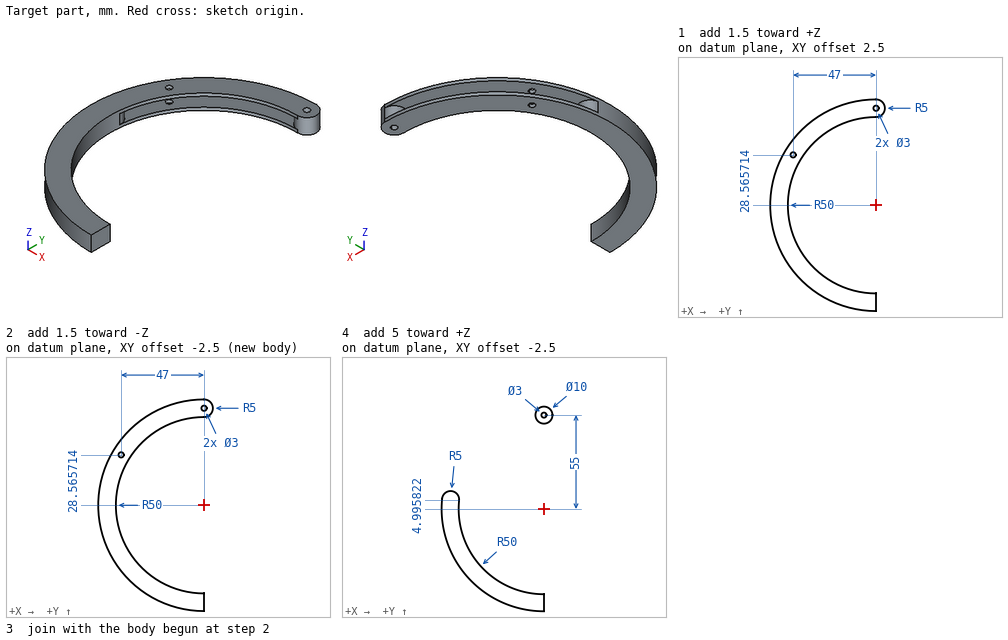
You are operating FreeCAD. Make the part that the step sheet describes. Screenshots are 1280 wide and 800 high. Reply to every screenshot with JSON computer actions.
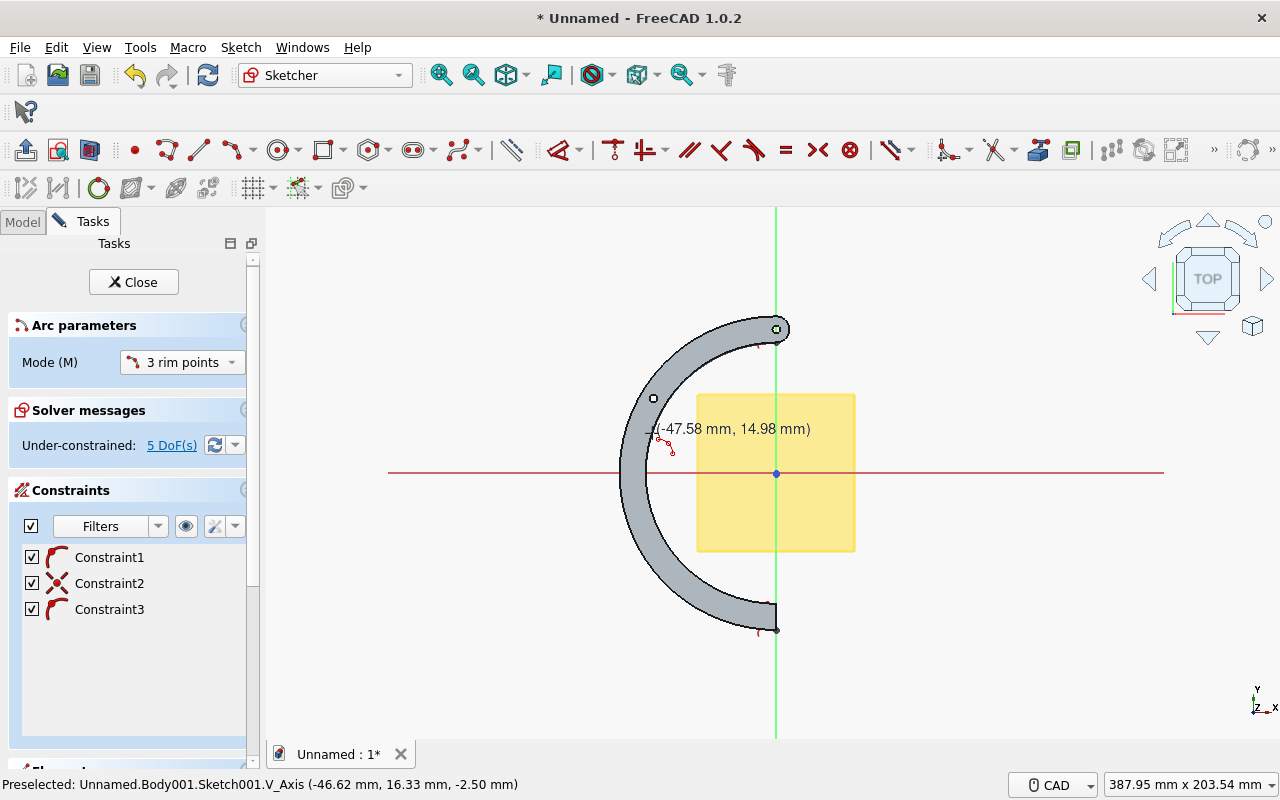
{"action": "left_click", "coordinate": [776, 343]}
{"action": "left_click", "coordinate": [776, 316]}
{"action": "left_click", "coordinate": [789, 329]}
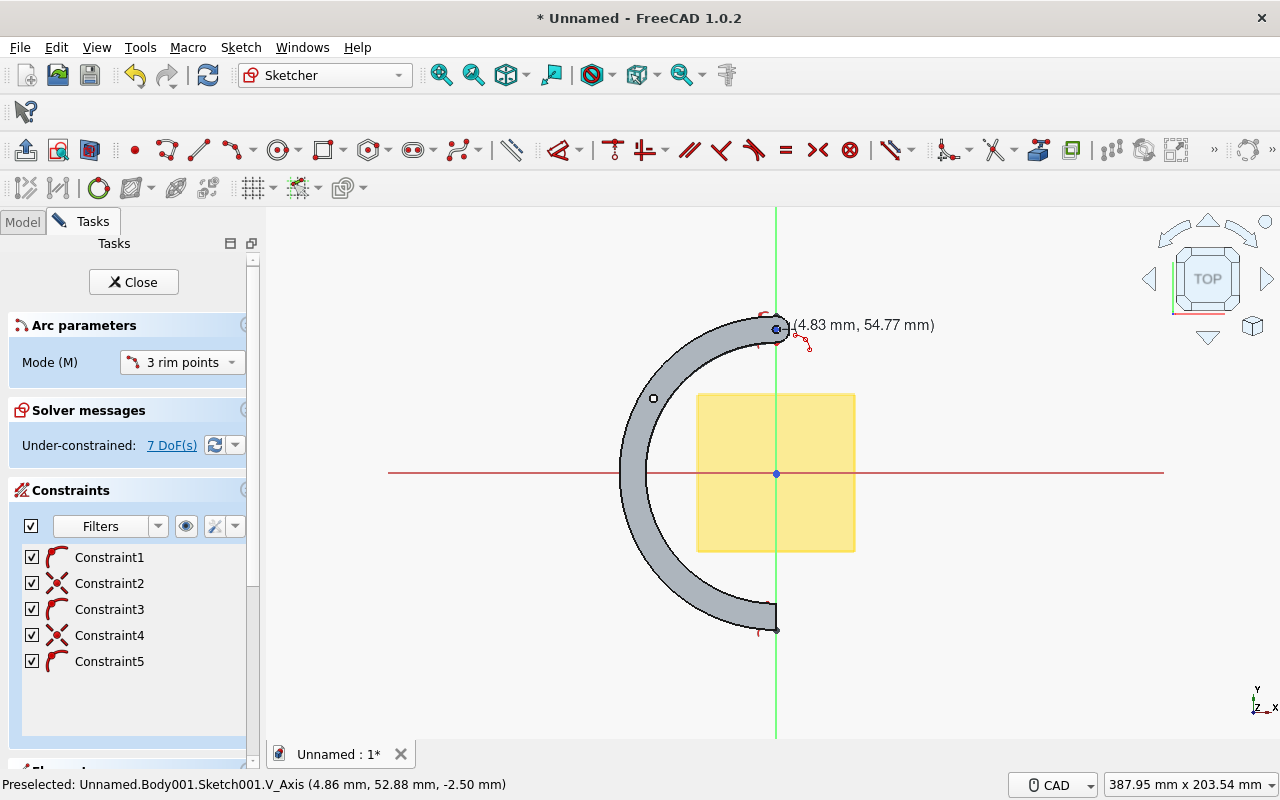
{"action": "left_click", "coordinate": [776, 317]}
{"action": "left_click", "coordinate": [776, 631]}
{"action": "left_click", "coordinate": [627, 425]}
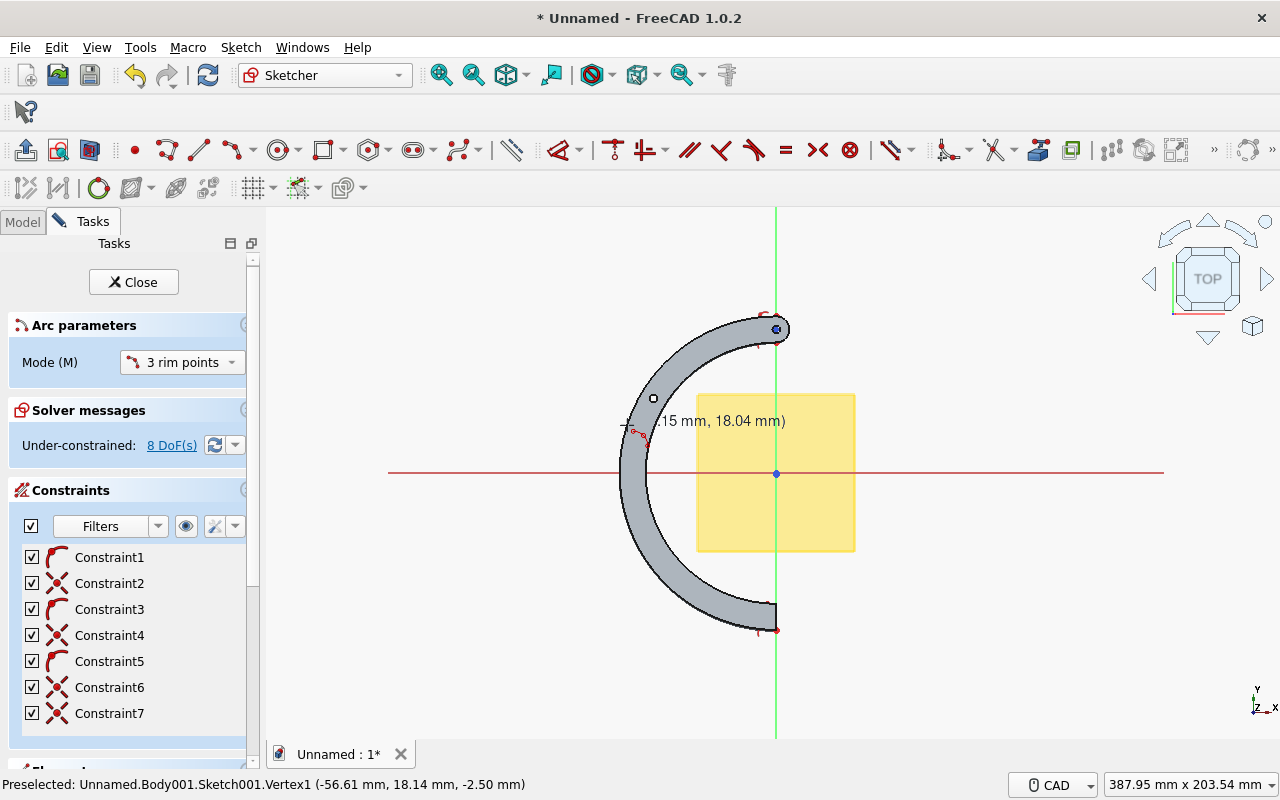
{"action": "left_click", "coordinate": [278, 150]}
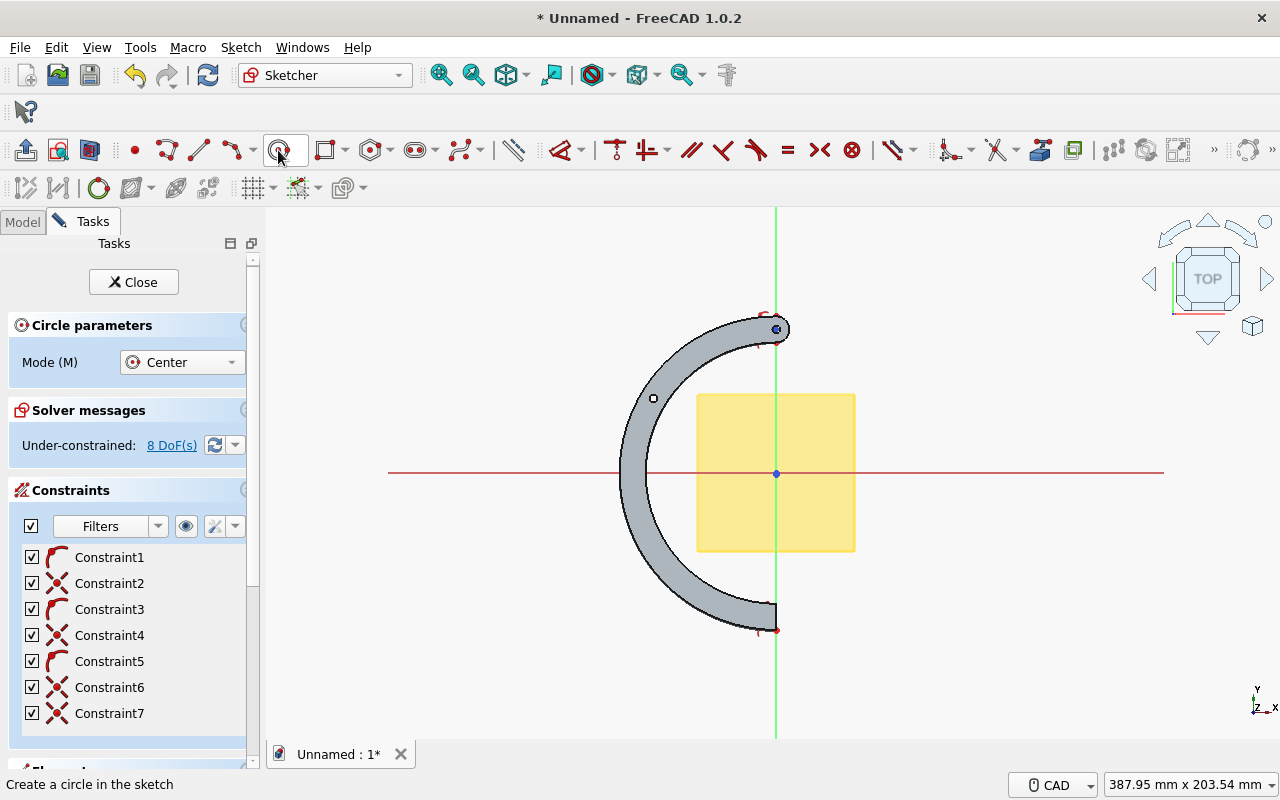
{"action": "scroll", "coordinate": [654, 399], "scroll_direction": "up", "scroll_amount": 9}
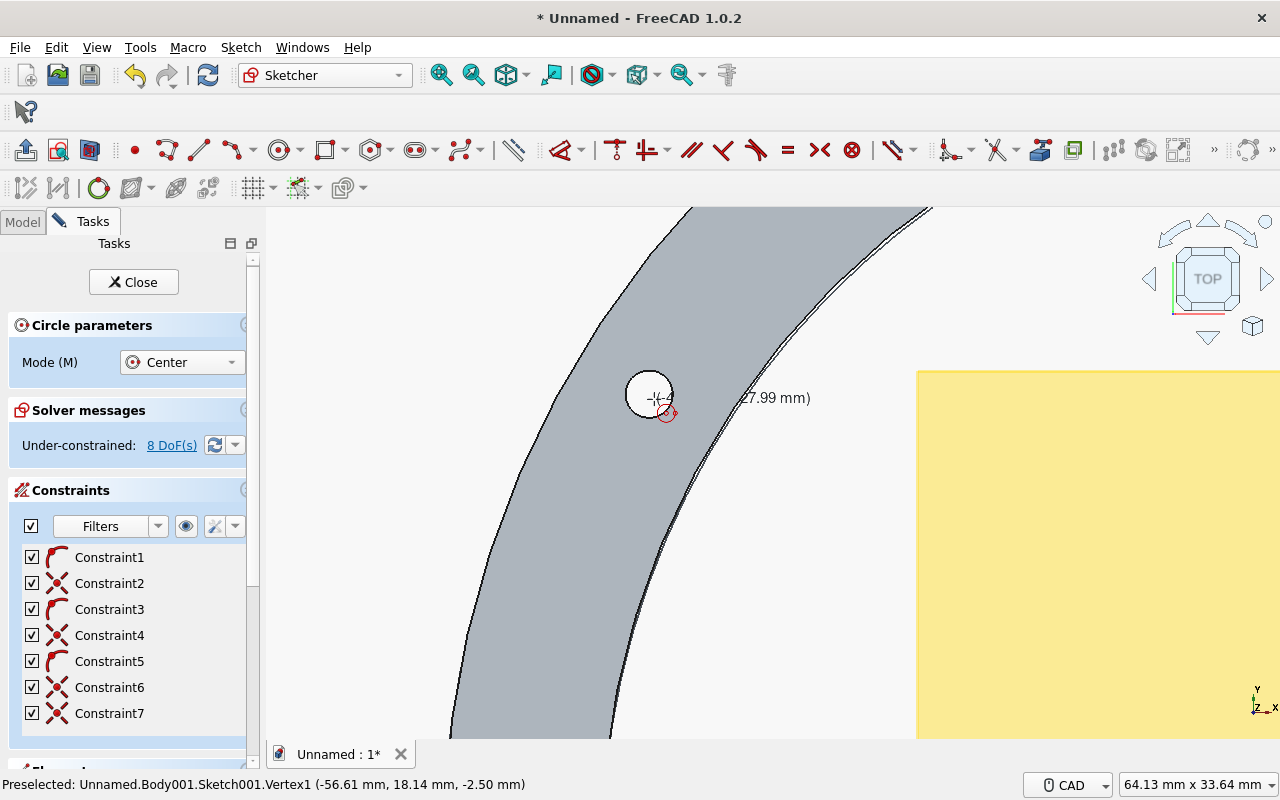
{"action": "scroll", "coordinate": [654, 399], "scroll_direction": "down", "scroll_amount": 9}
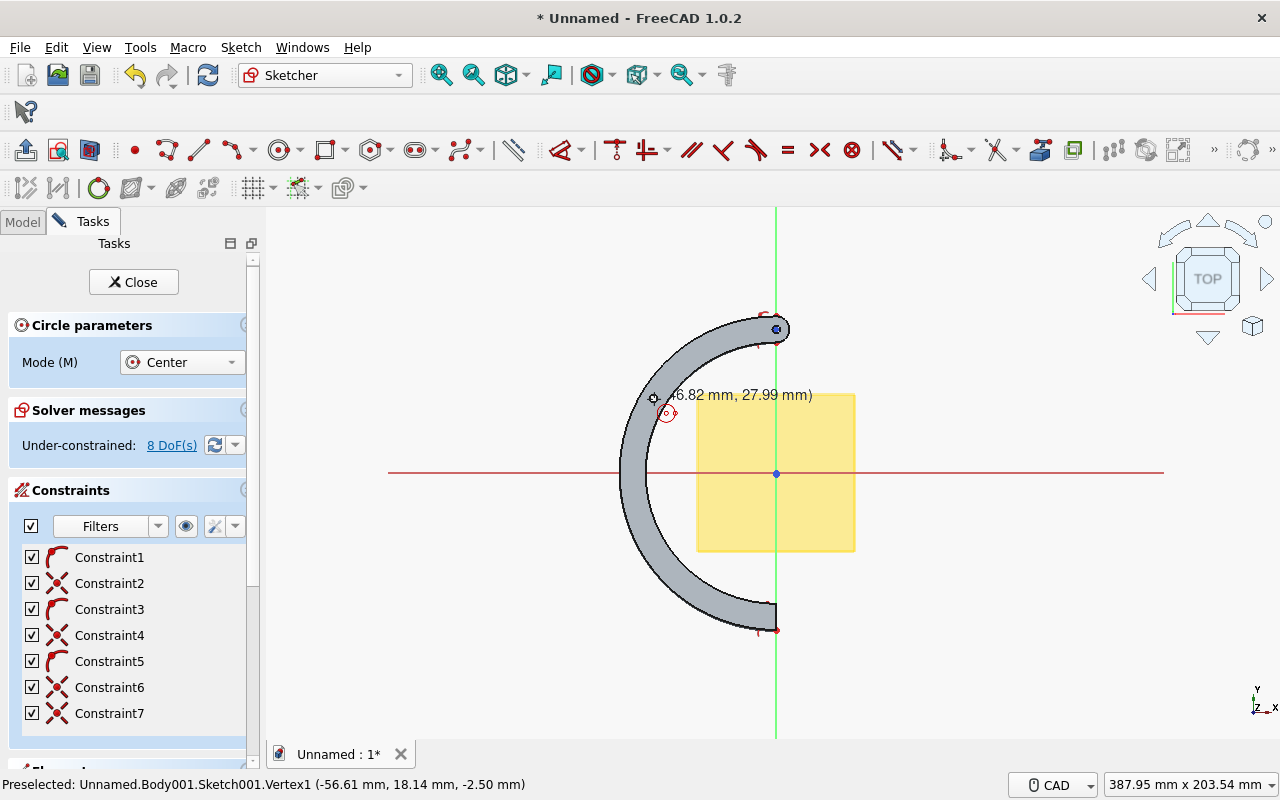
{"action": "left_click", "coordinate": [654, 399]}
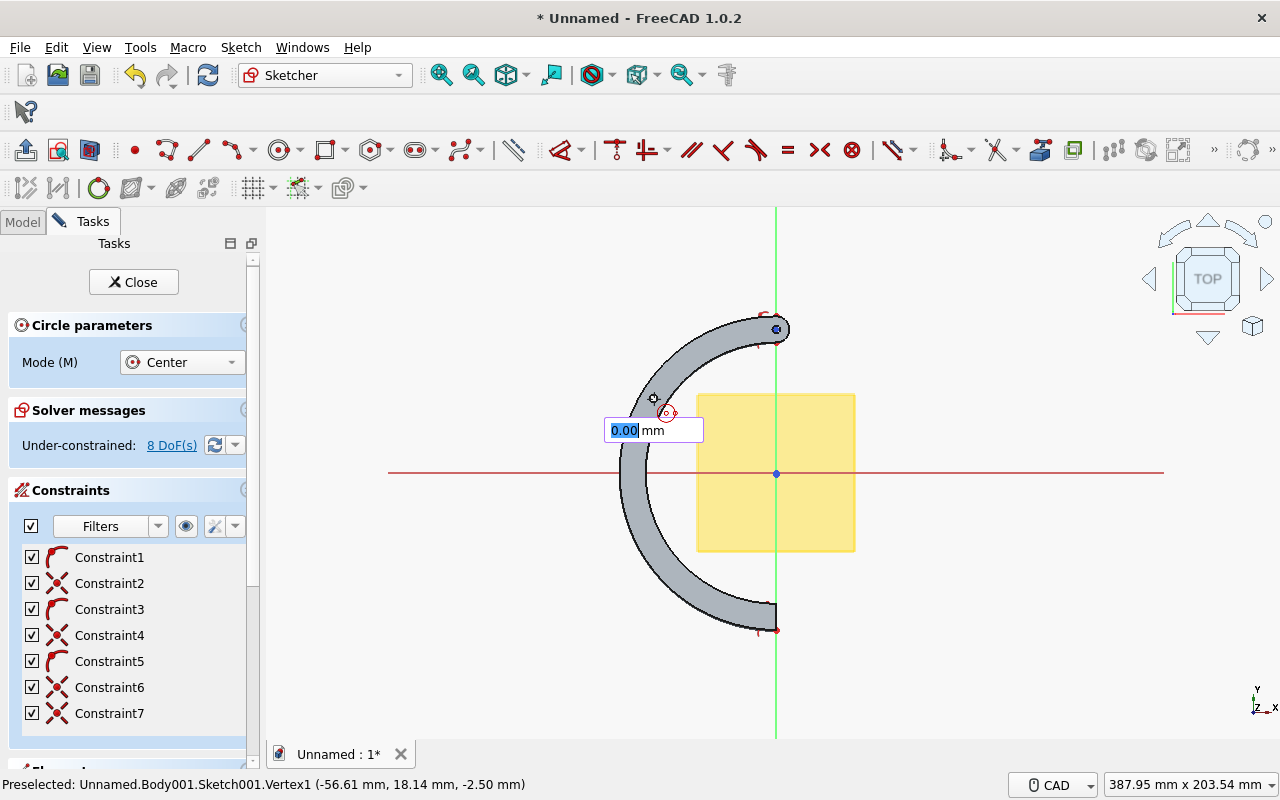
{"action": "scroll", "coordinate": [652, 402], "scroll_direction": "up", "scroll_amount": 7}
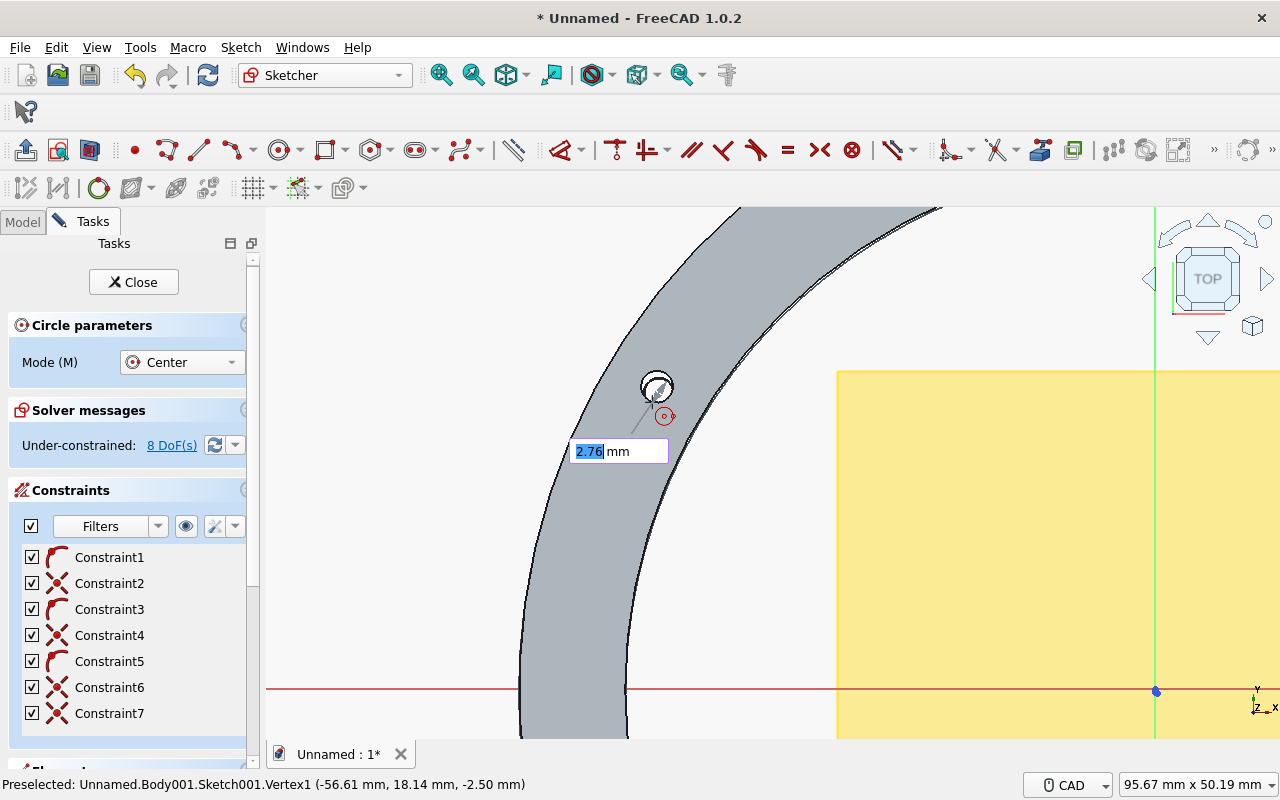
{"action": "left_click", "coordinate": [652, 402]}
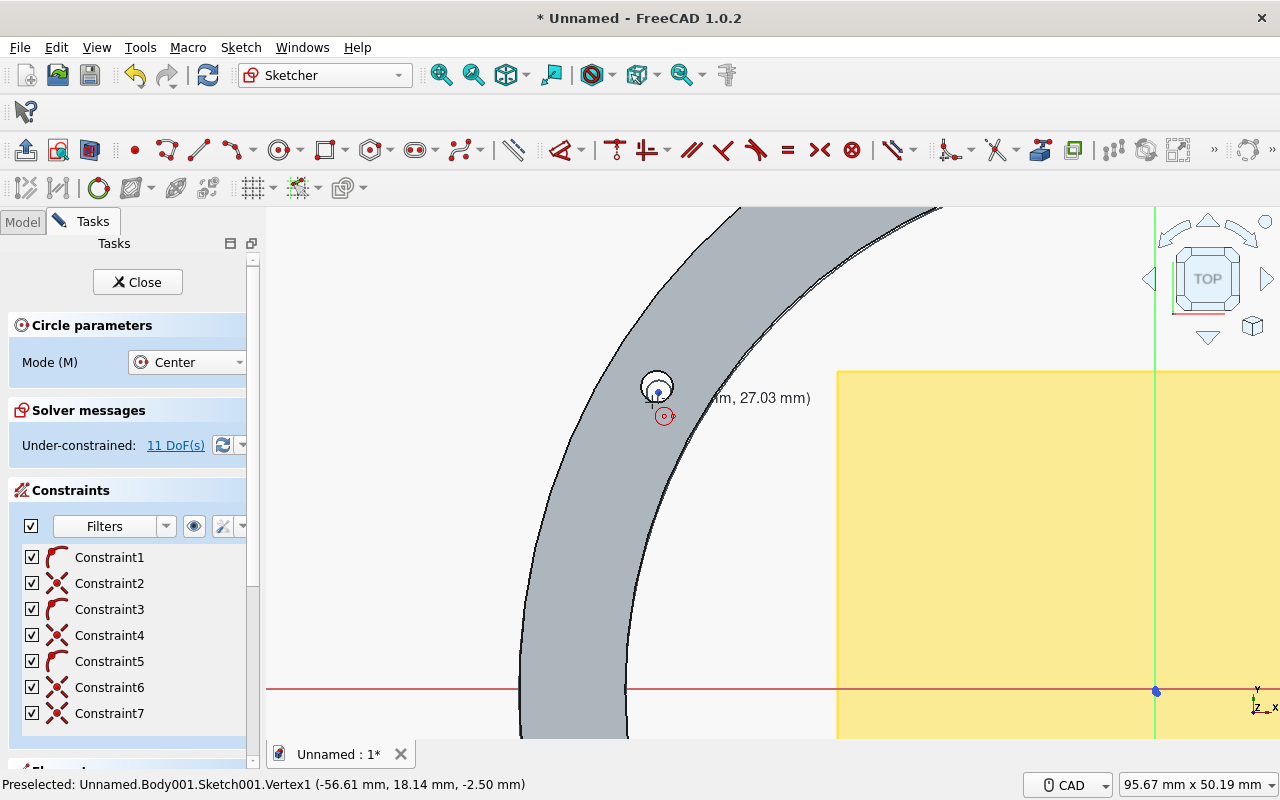
{"action": "scroll", "coordinate": [652, 402], "scroll_direction": "down", "scroll_amount": 7}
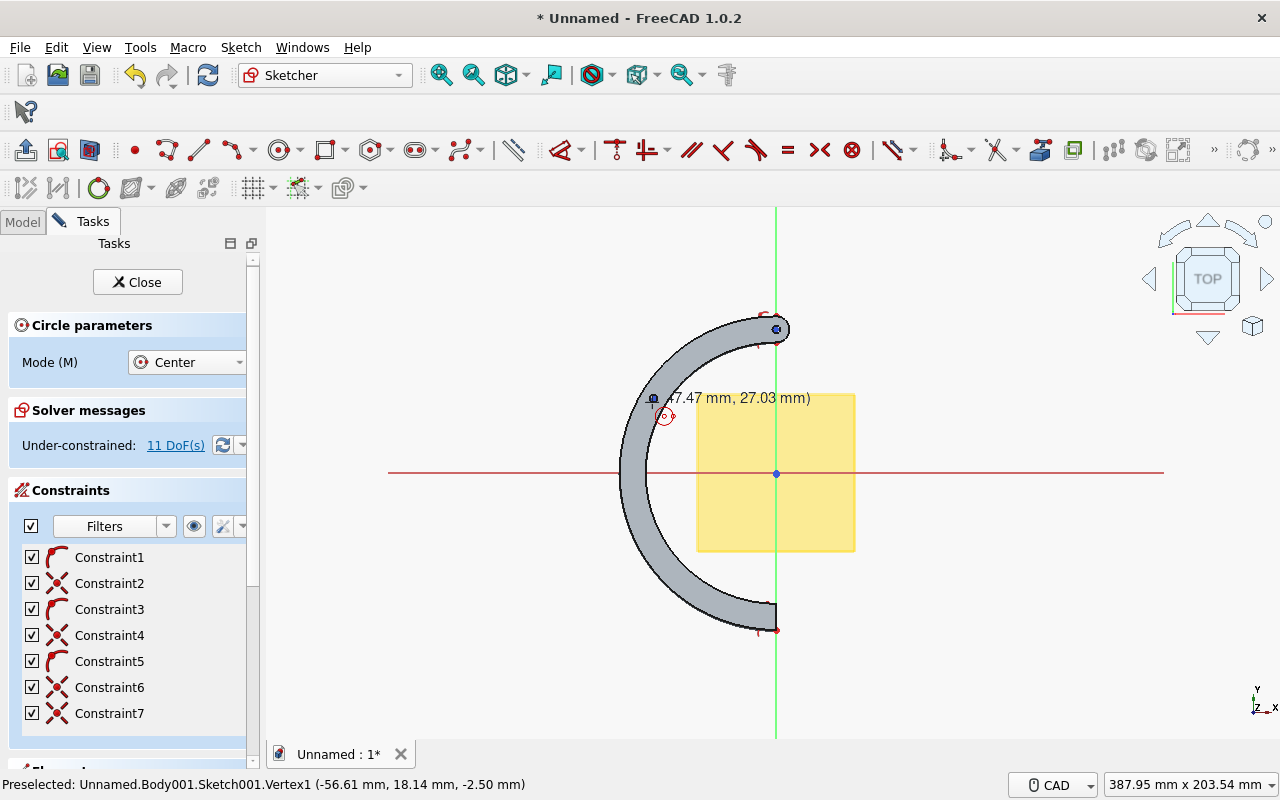
{"action": "scroll", "coordinate": [776, 329], "scroll_direction": "up", "scroll_amount": 9}